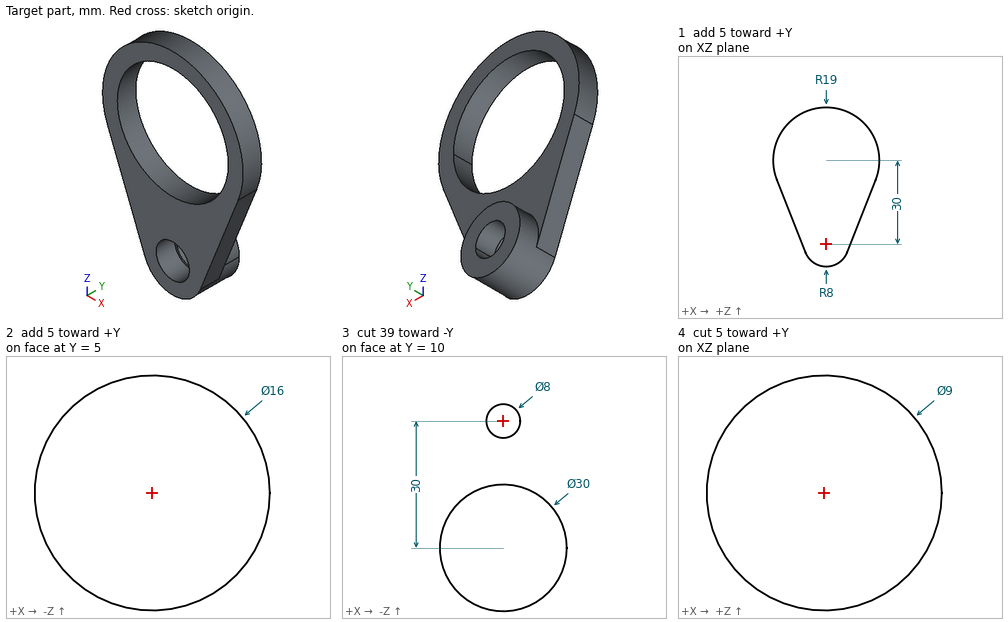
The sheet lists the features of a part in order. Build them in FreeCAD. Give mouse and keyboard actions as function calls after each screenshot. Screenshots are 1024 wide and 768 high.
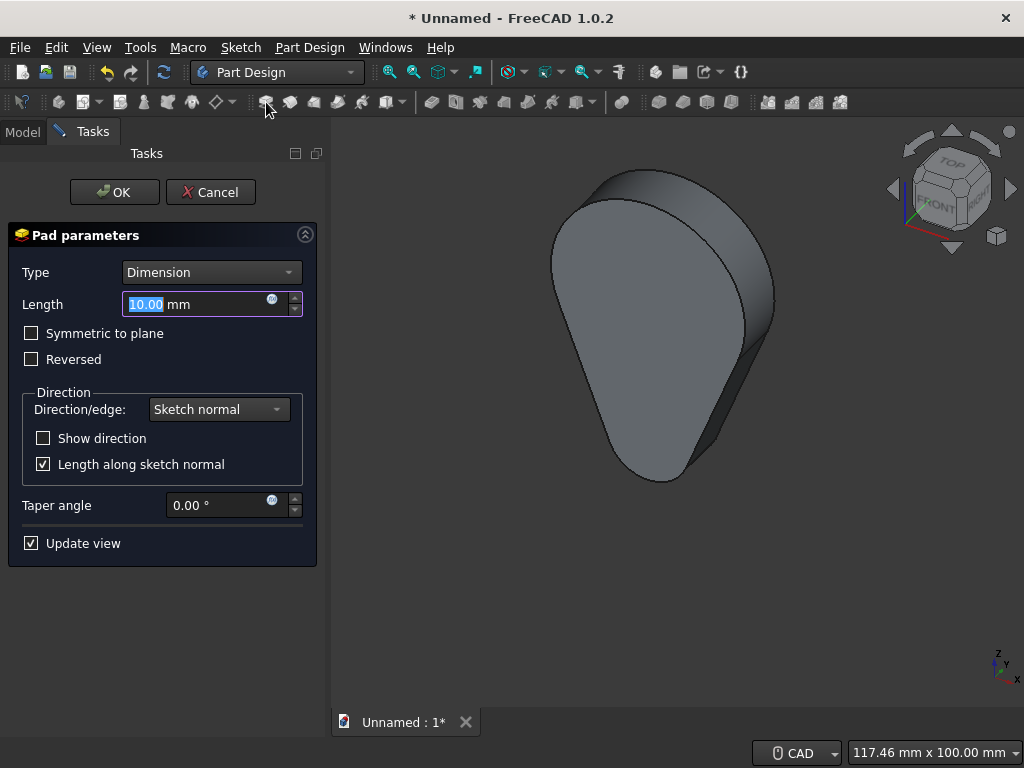
text(5)
key(Tab)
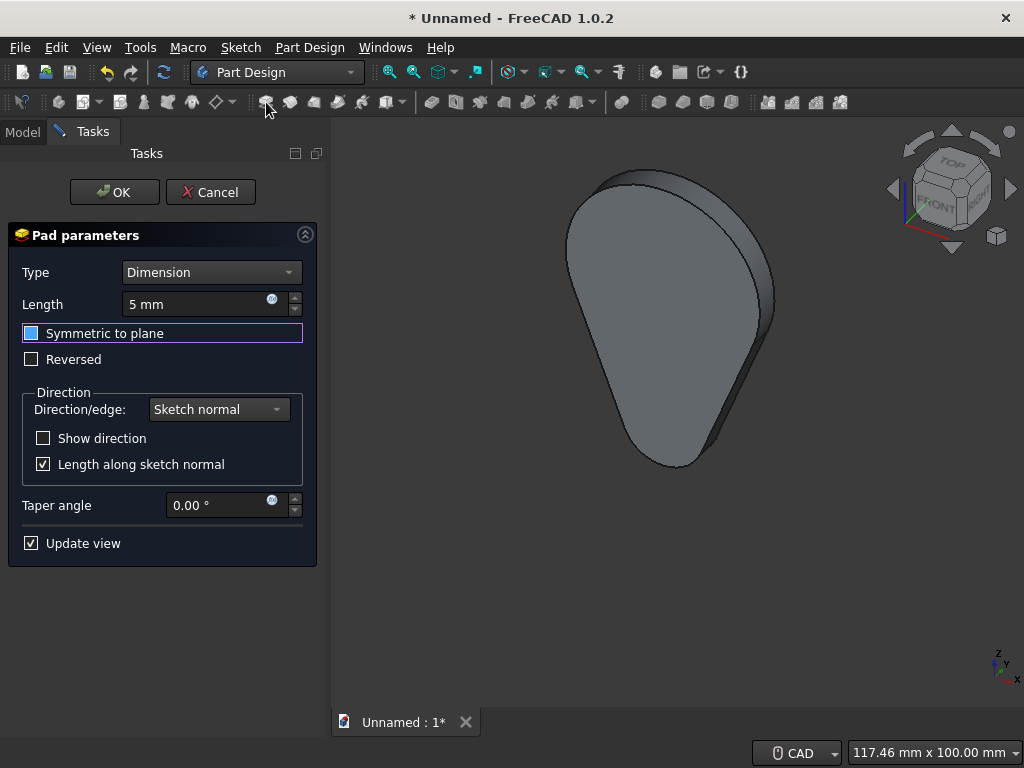
click(30, 359)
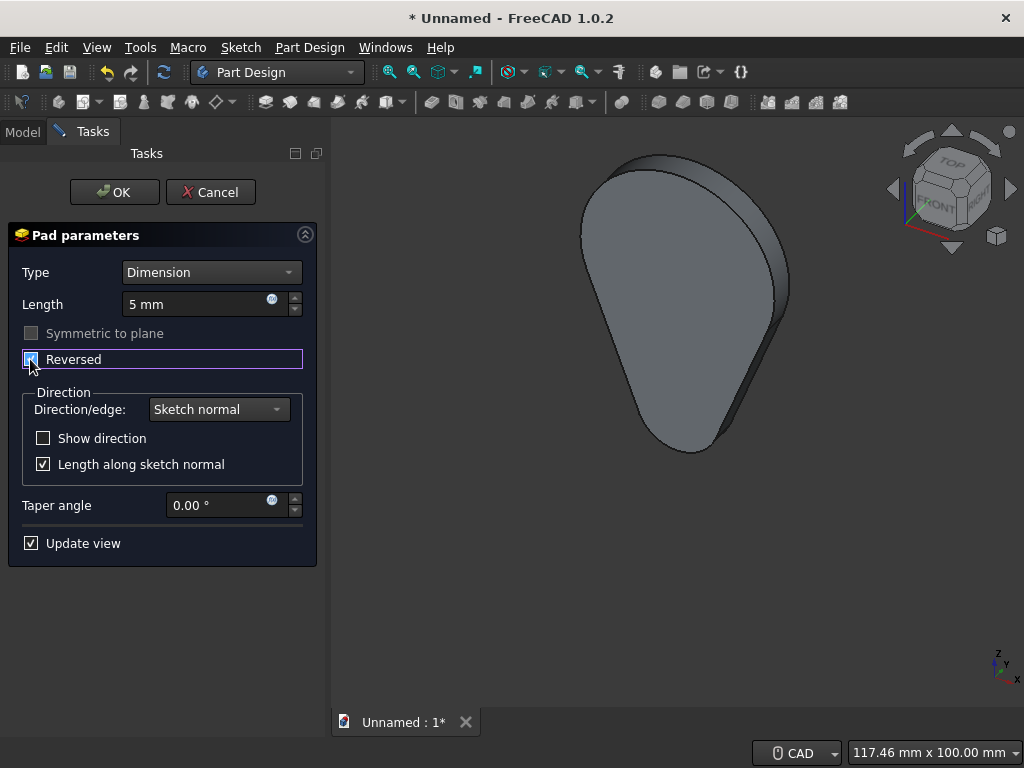
click(115, 192)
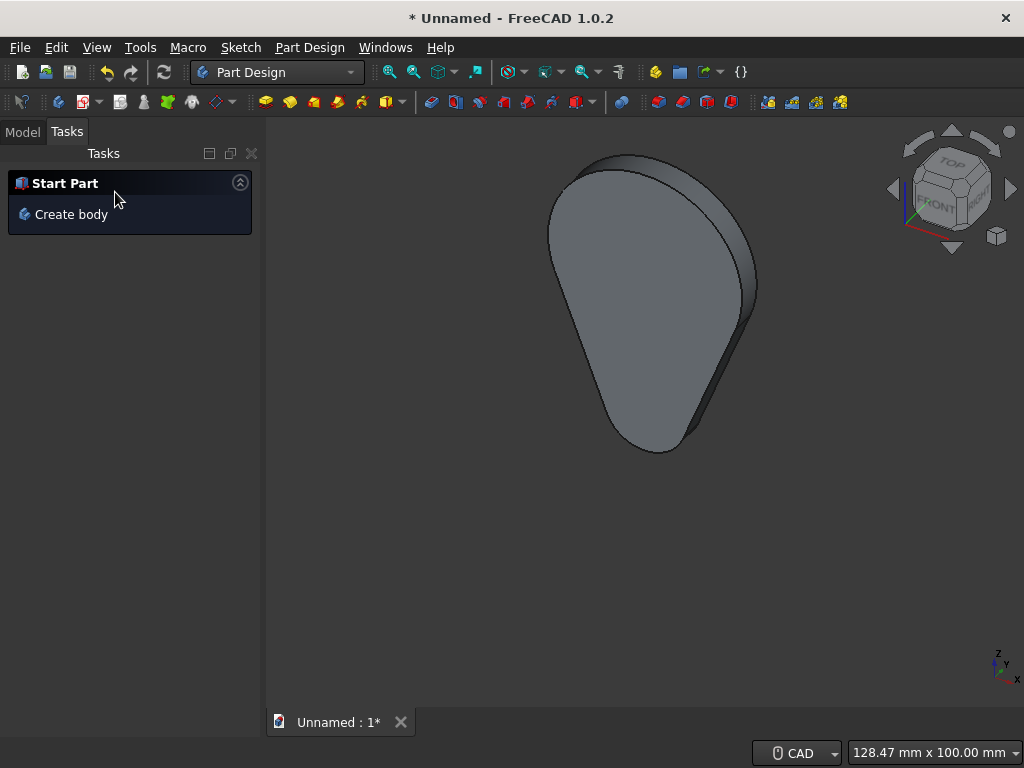
key(4)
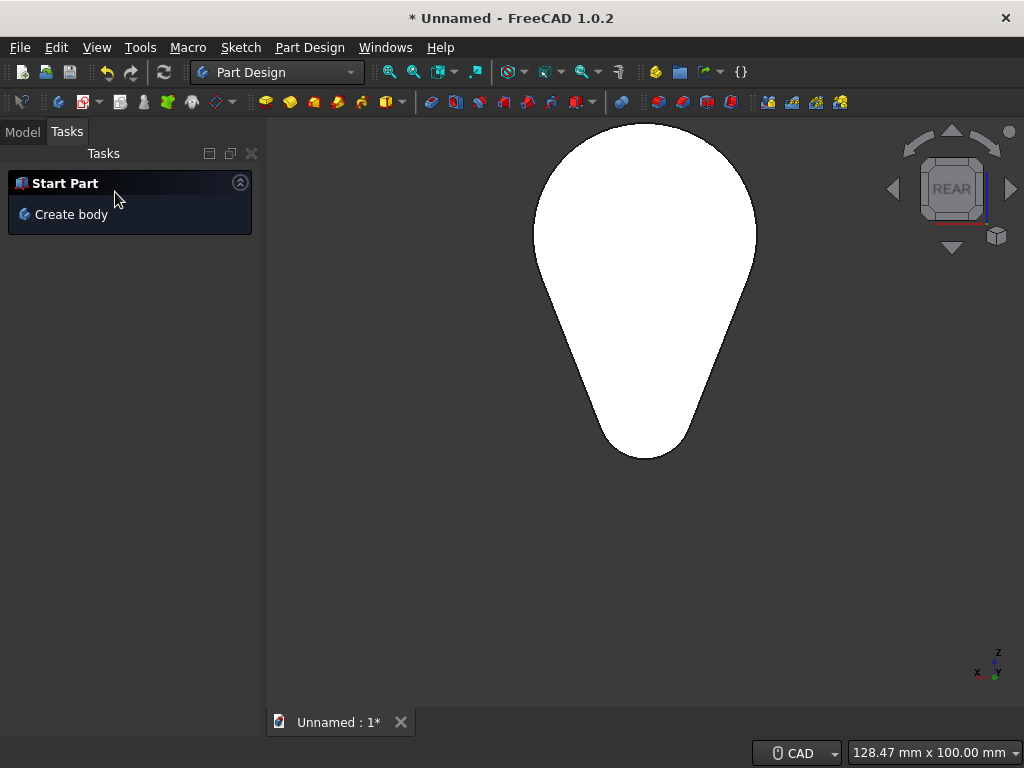
click(645, 242)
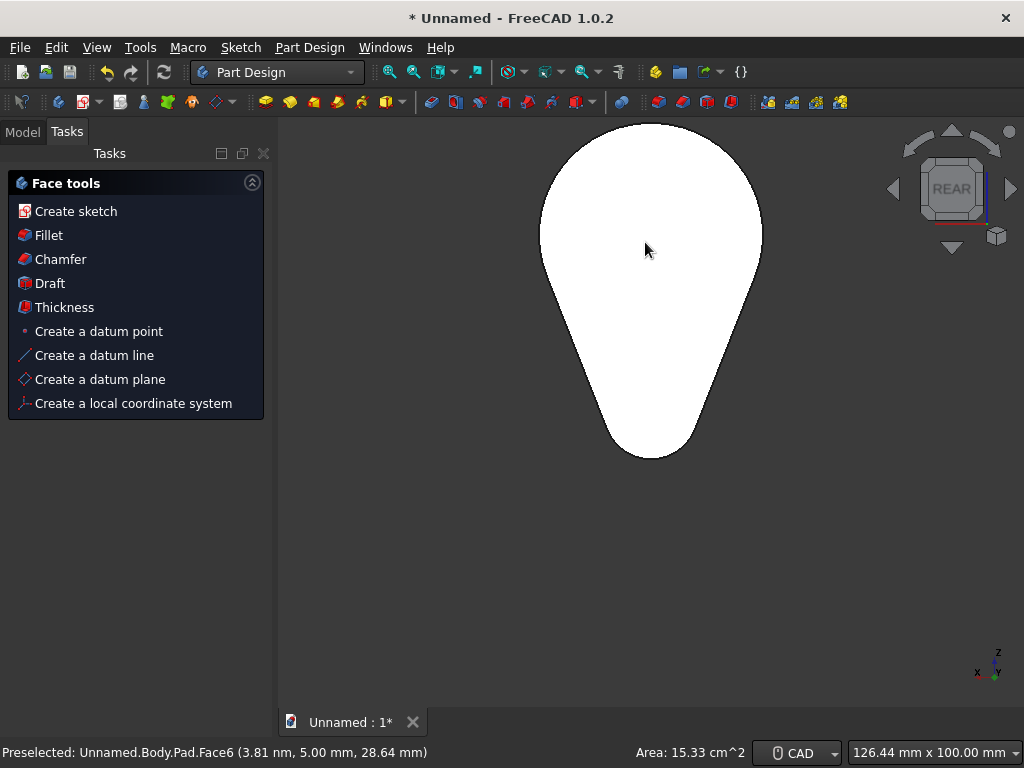
click(84, 102)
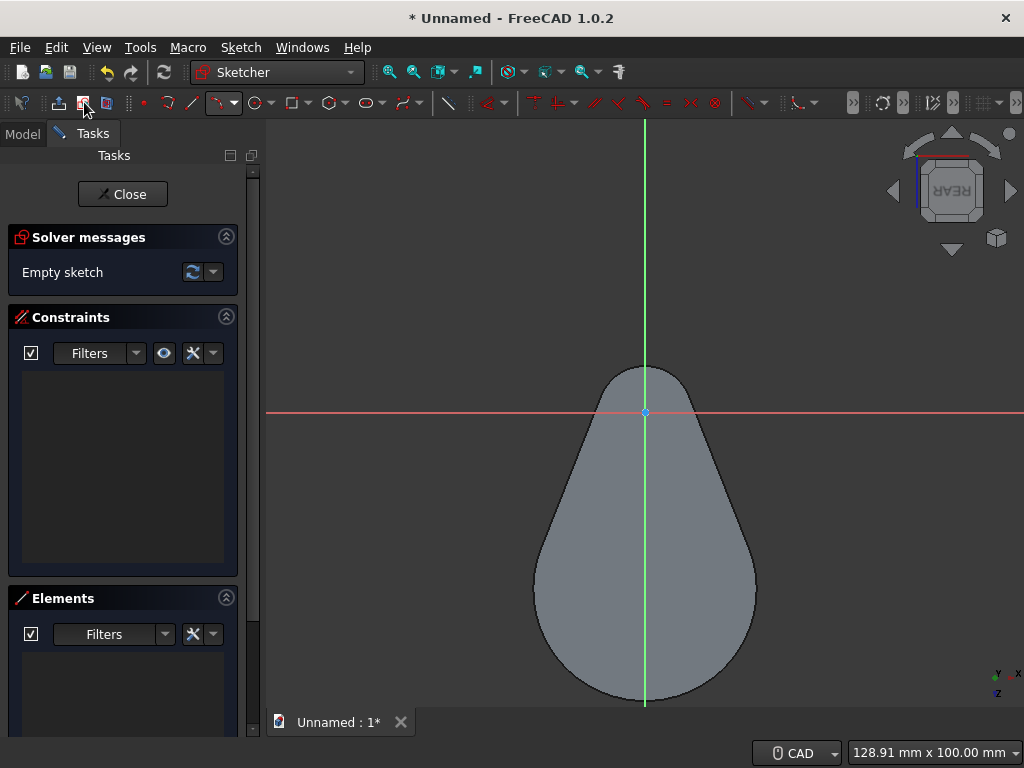
scroll(667, 413, up, 7)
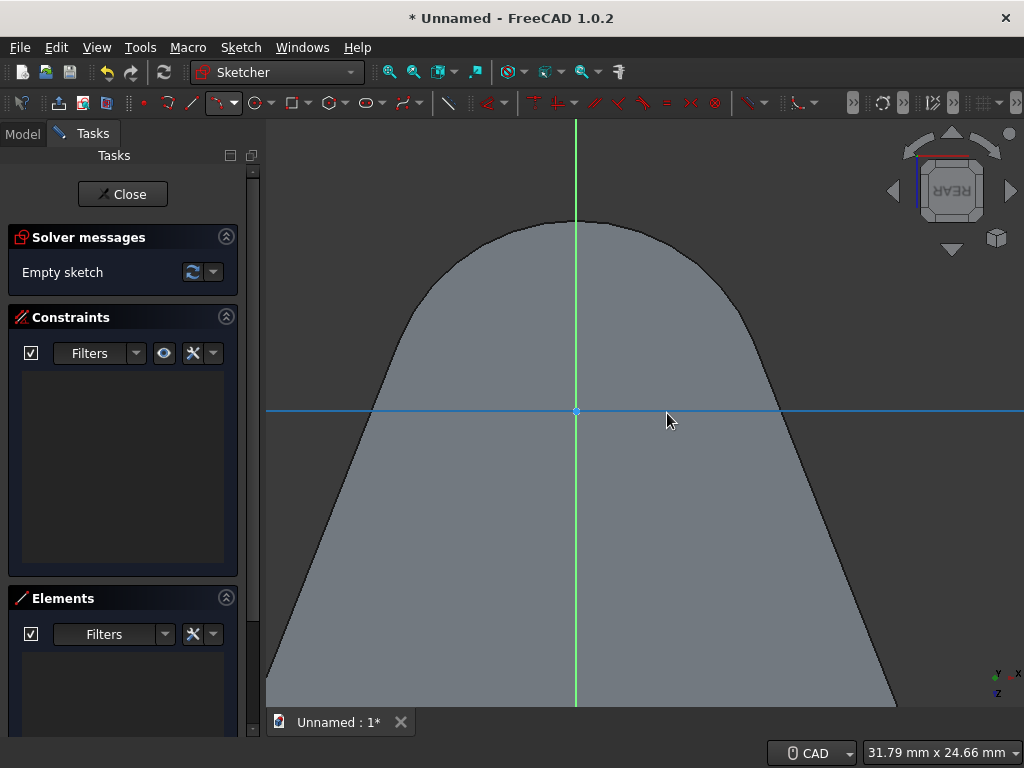
click(256, 104)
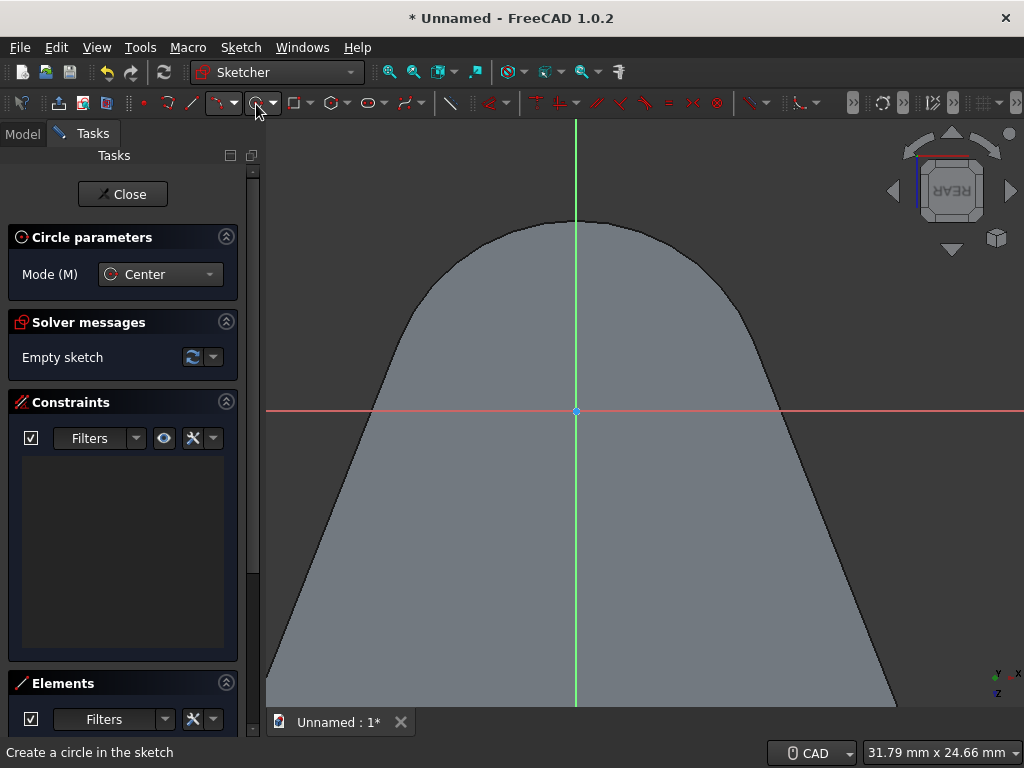
click(576, 411)
move(711, 277)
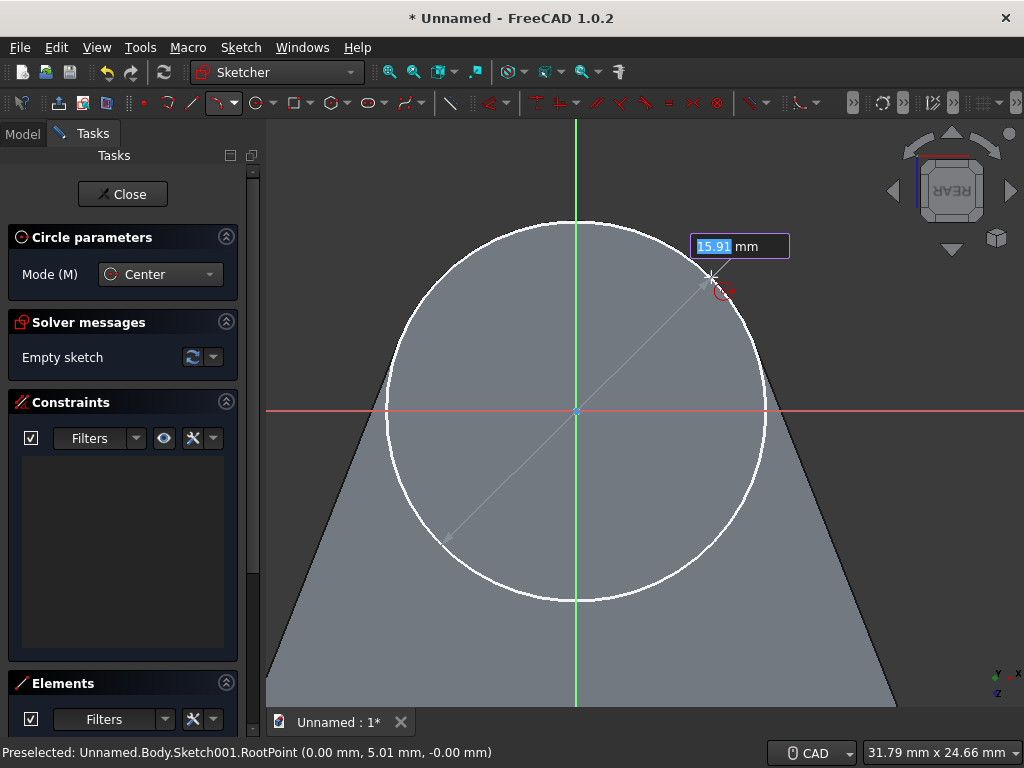
text(16)
key(Return)
key(Escape)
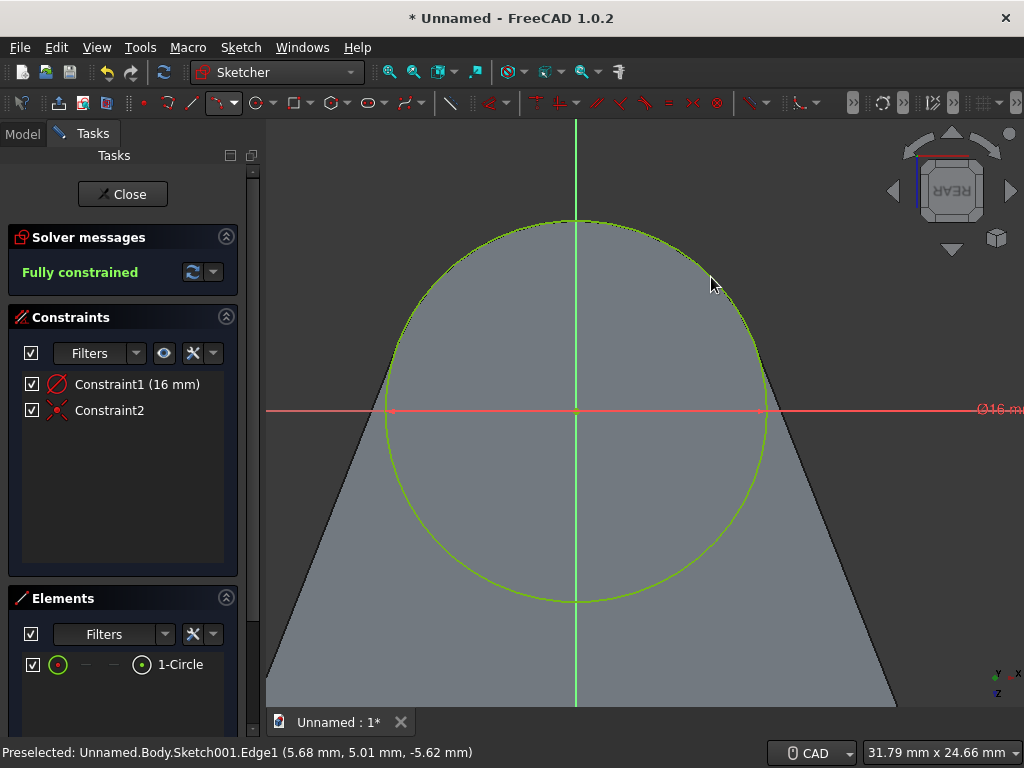
click(123, 194)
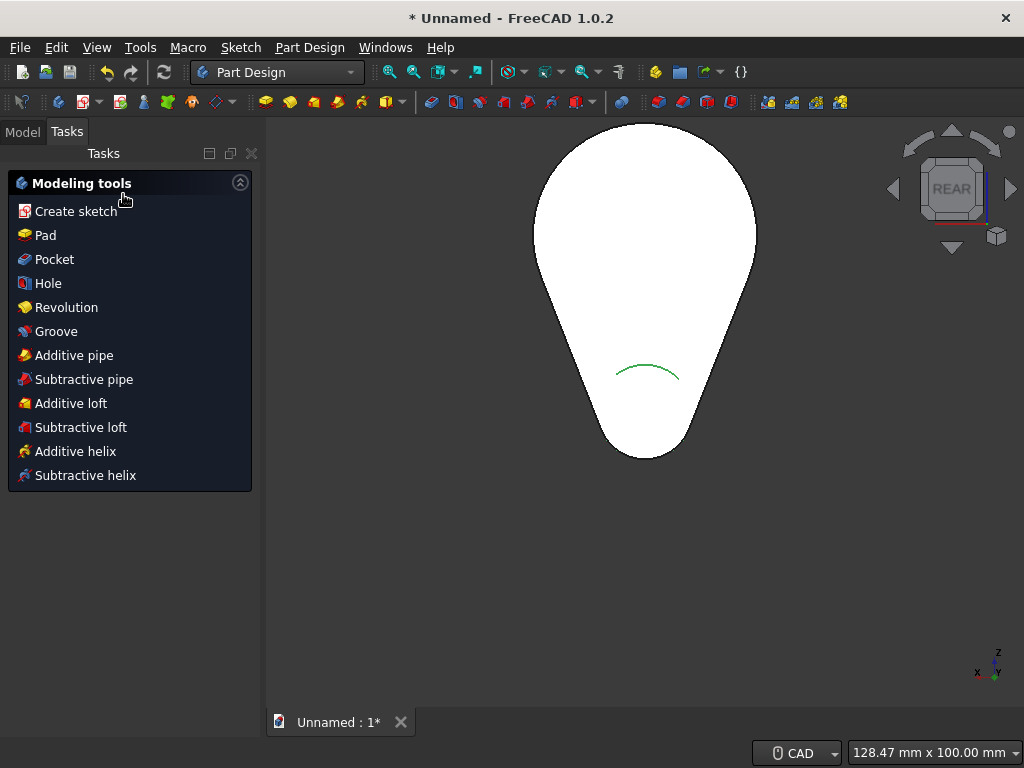
click(266, 102)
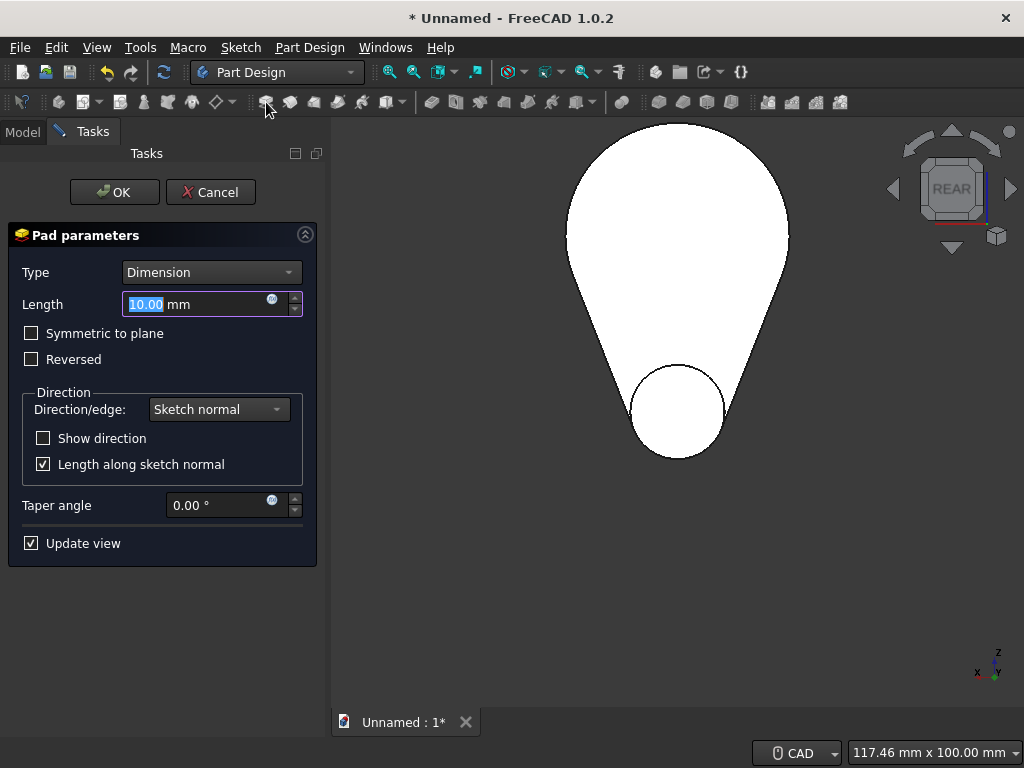
text(5)
key(Tab)